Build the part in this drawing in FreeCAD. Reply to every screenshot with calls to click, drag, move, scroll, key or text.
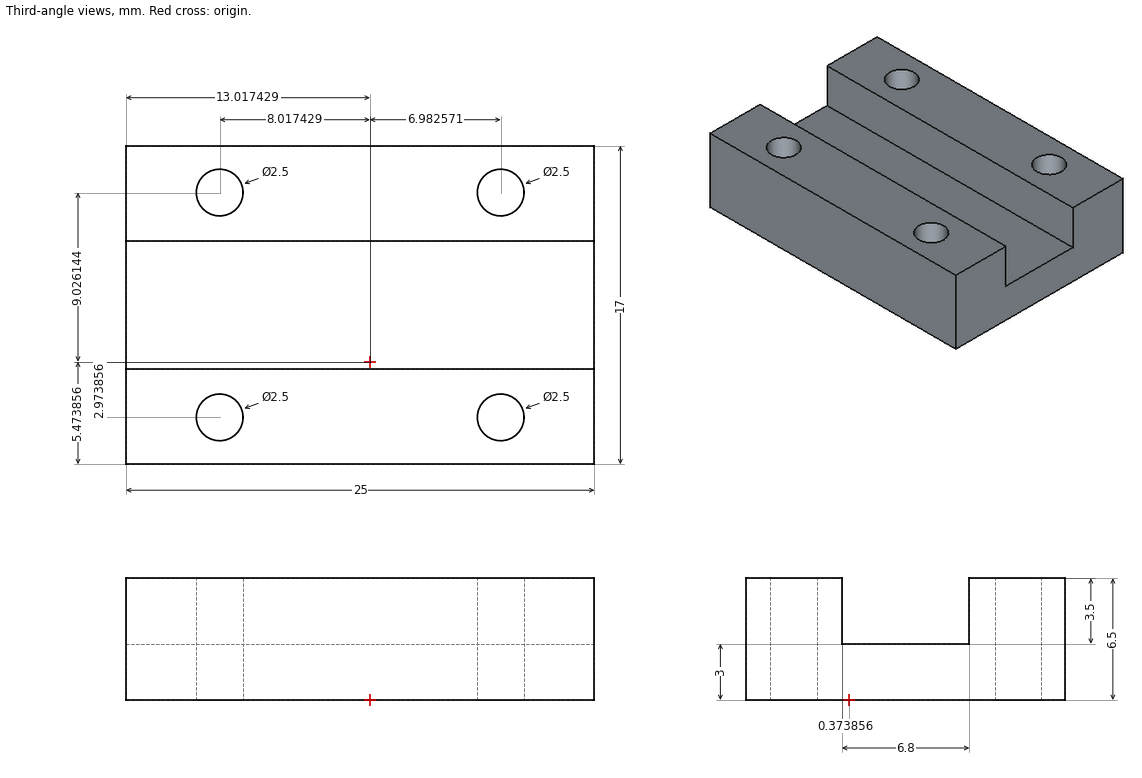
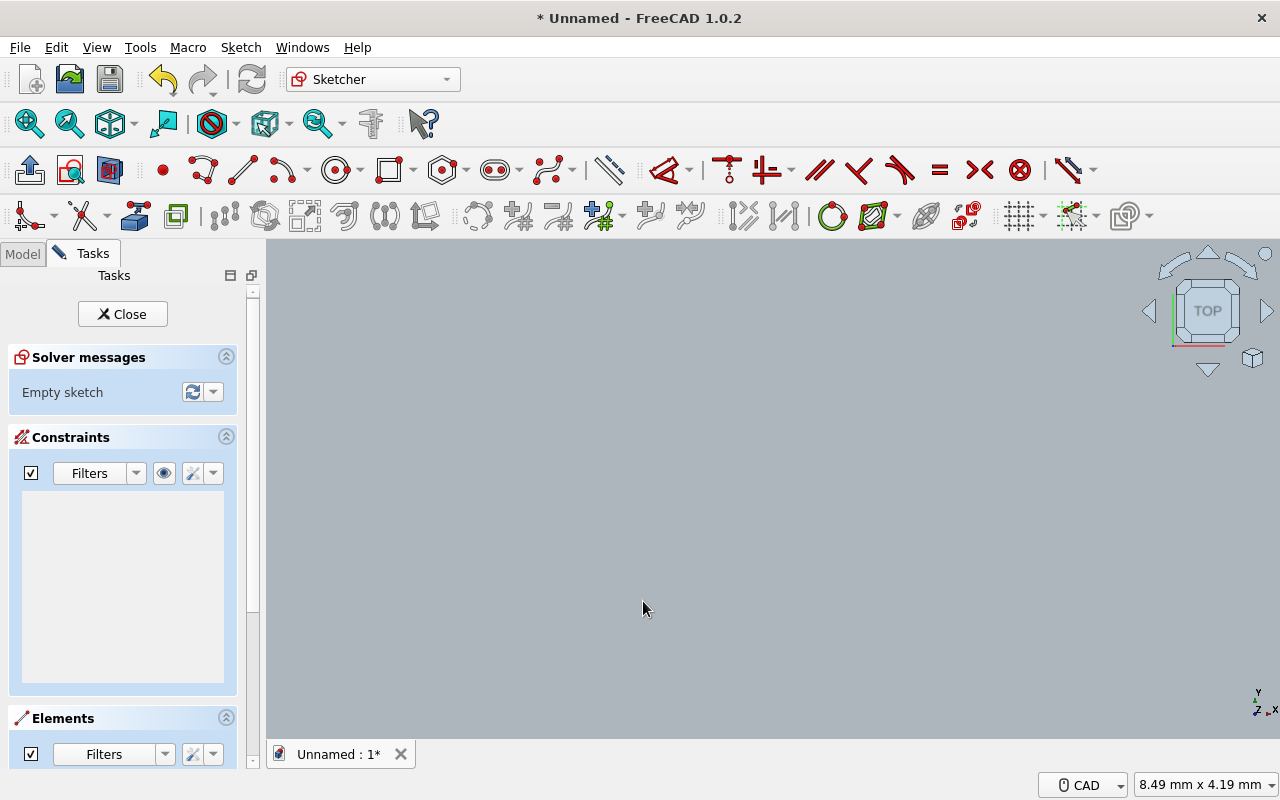
key(g)
key(c)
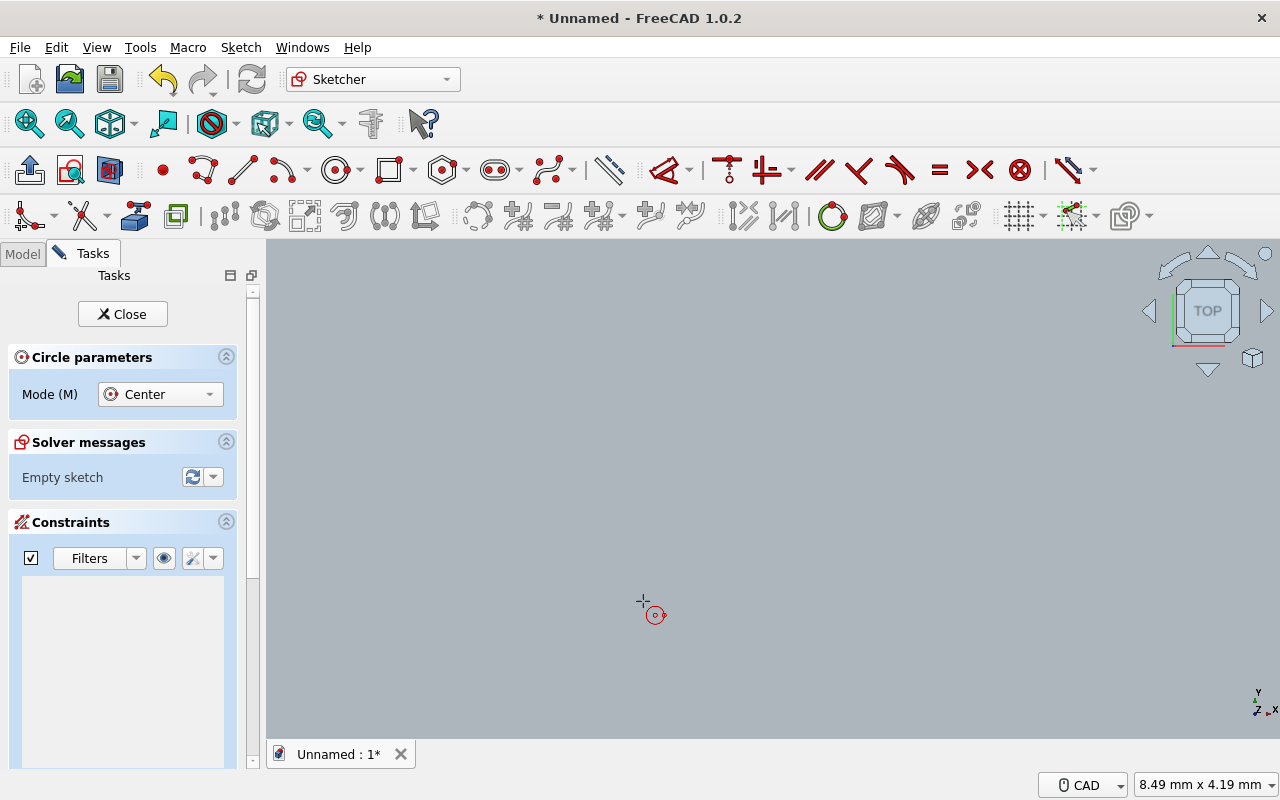
click(705, 486)
move(811, 380)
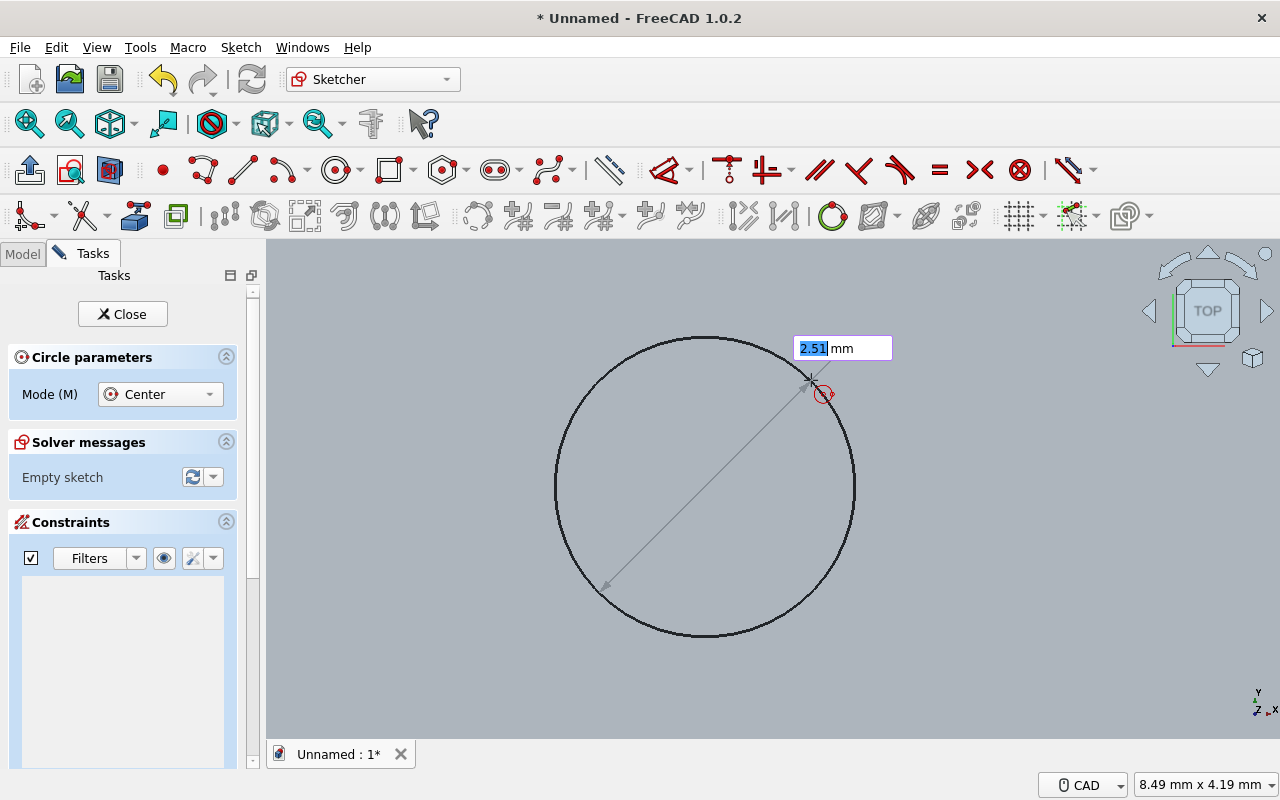
text(2.5)
key(Return)
key(Escape)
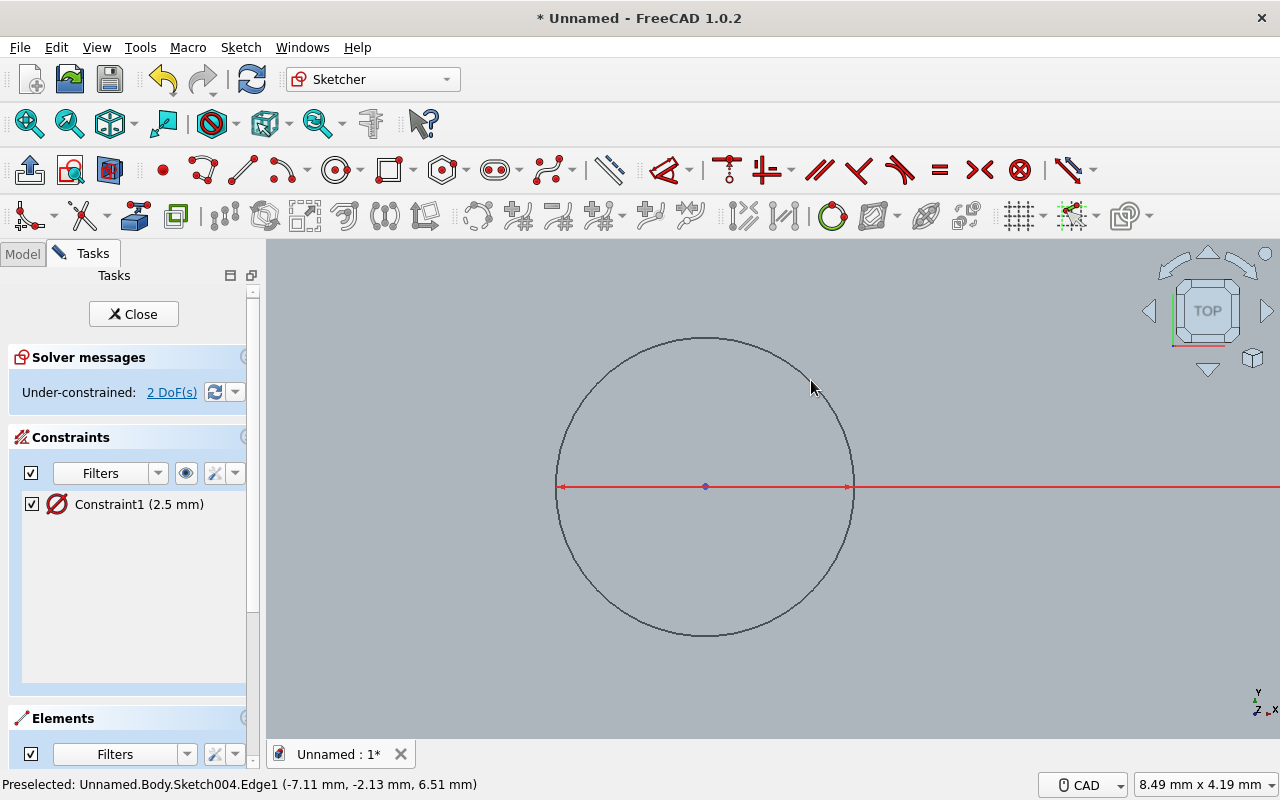
click(664, 170)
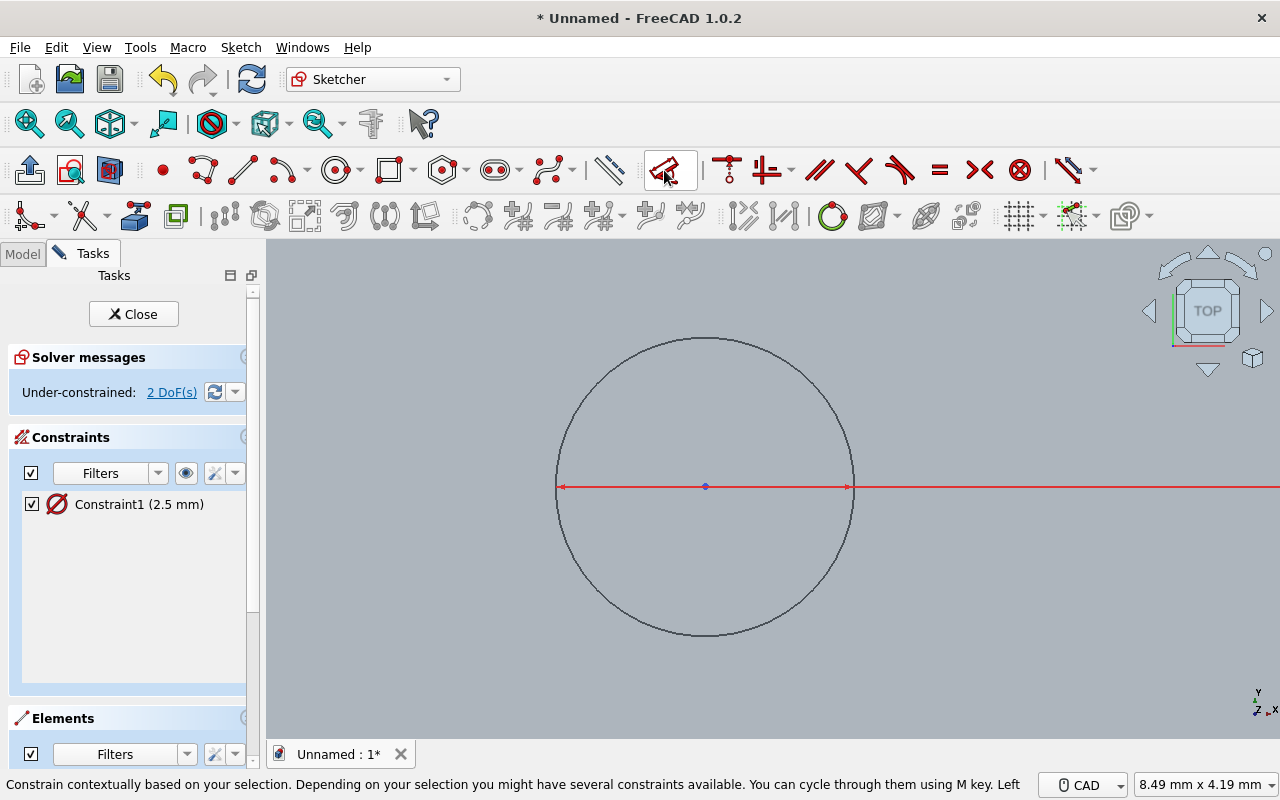
click(705, 487)
click(910, 521)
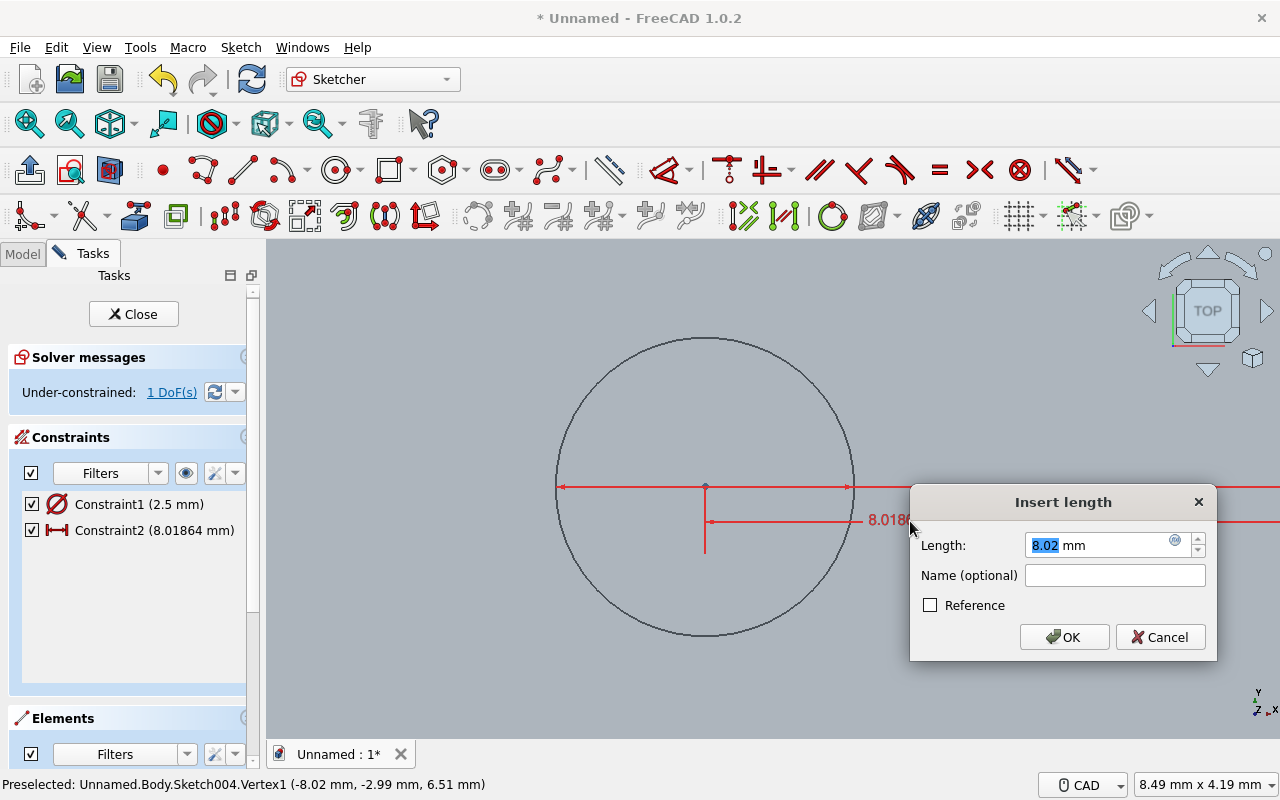
text(8.017429)
key(Return)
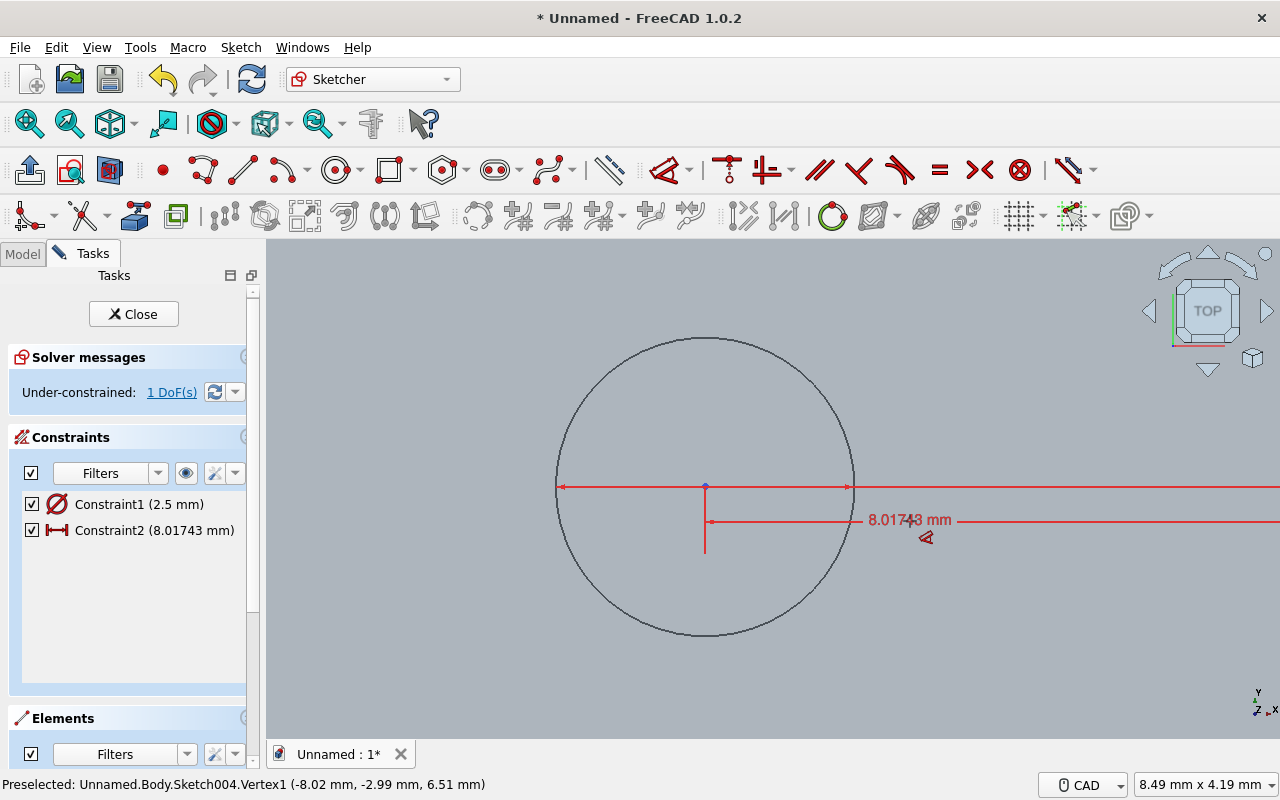
click(705, 487)
click(671, 377)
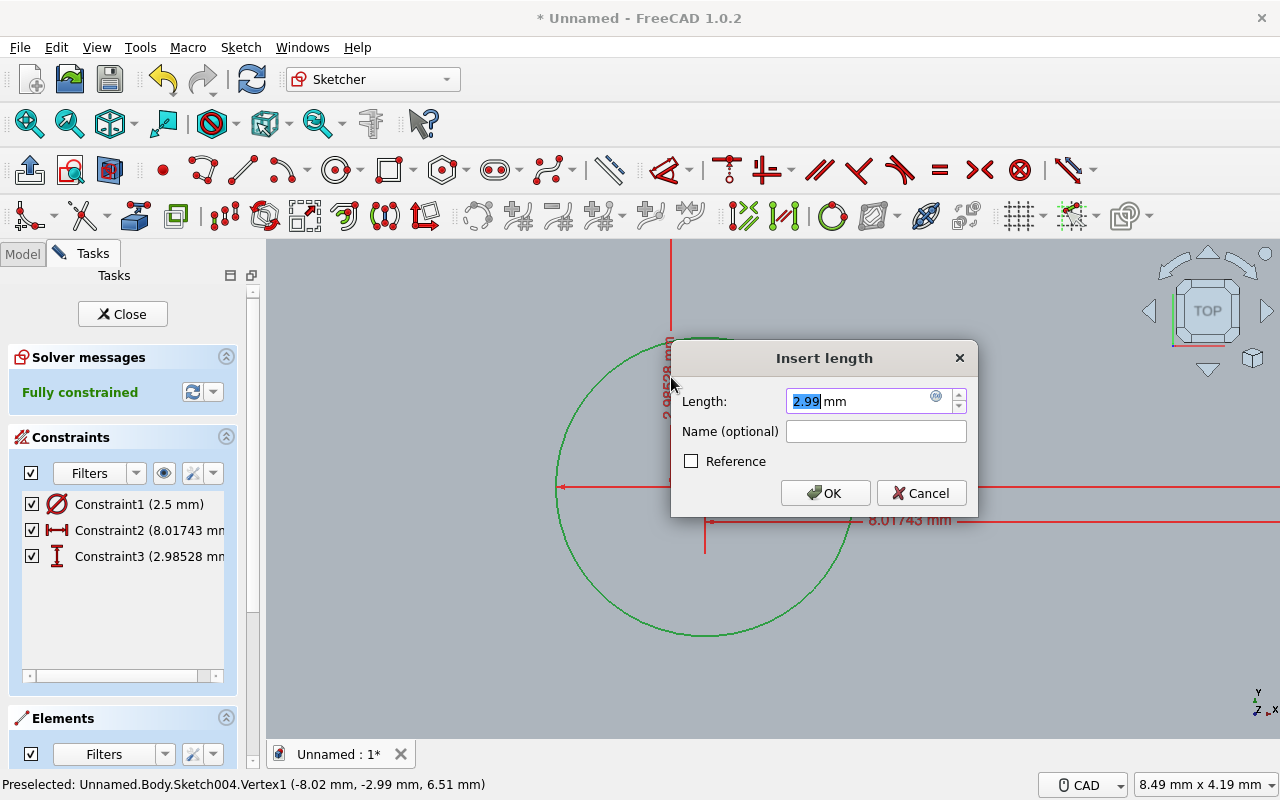
text(2.973856)
key(Return)
key(Escape)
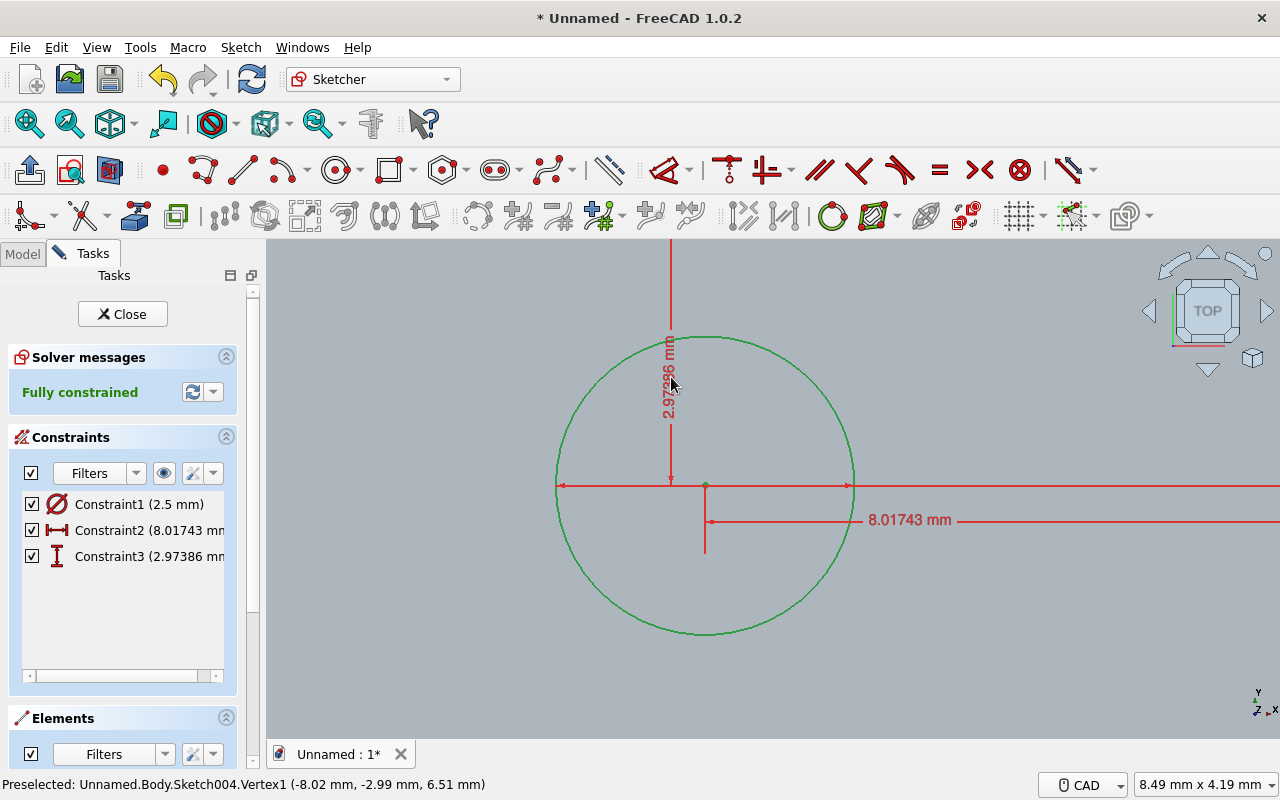
click(123, 314)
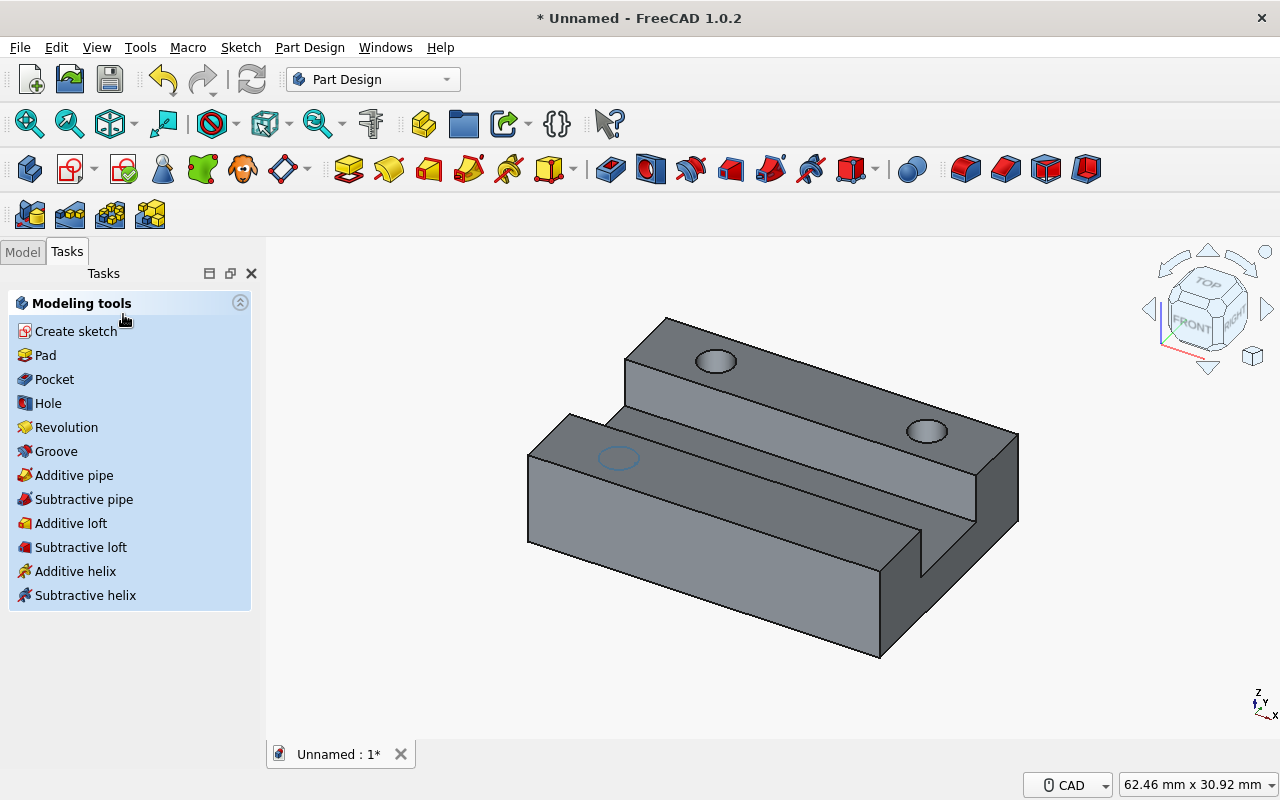
click(612, 170)